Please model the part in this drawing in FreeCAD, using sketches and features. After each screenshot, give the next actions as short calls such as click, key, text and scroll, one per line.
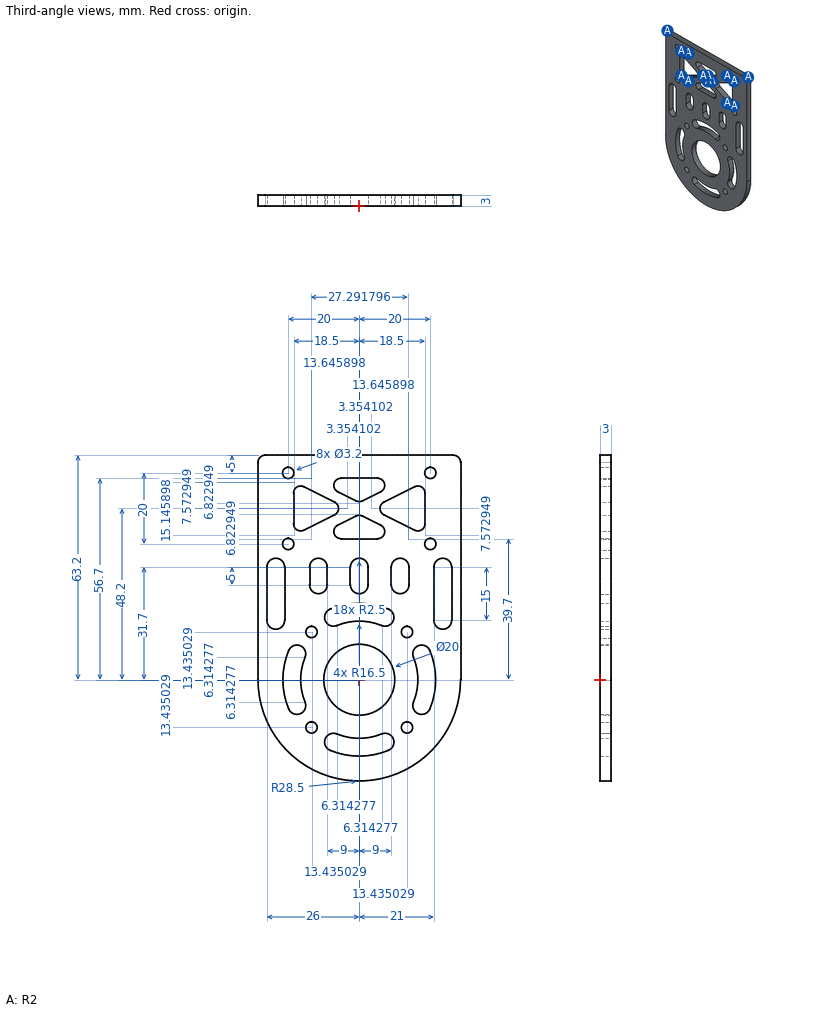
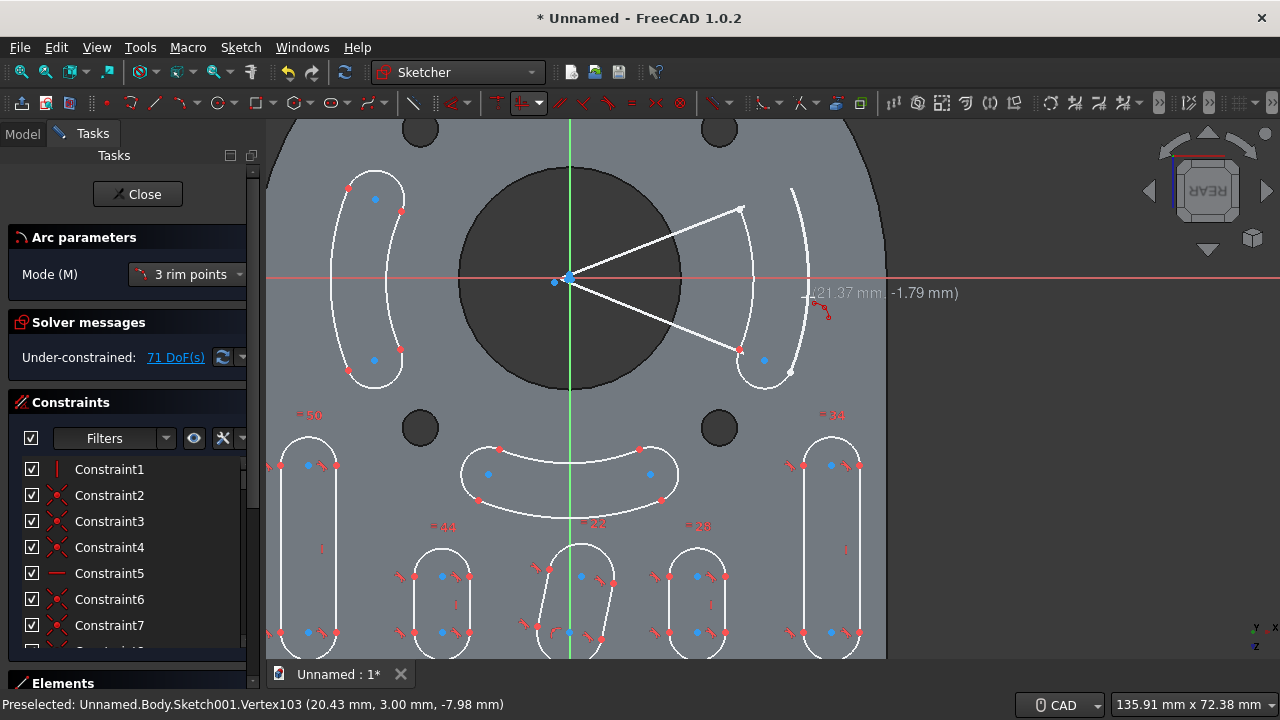
click(808, 297)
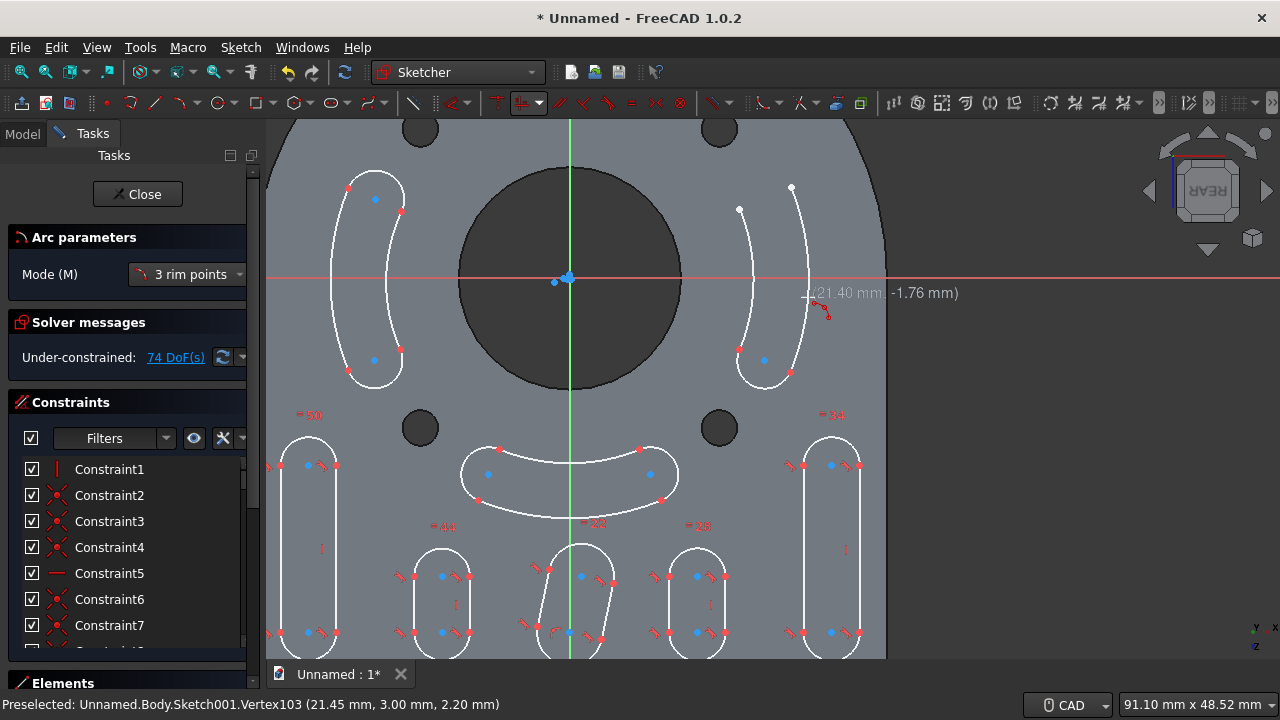
click(791, 188)
click(740, 209)
click(755, 172)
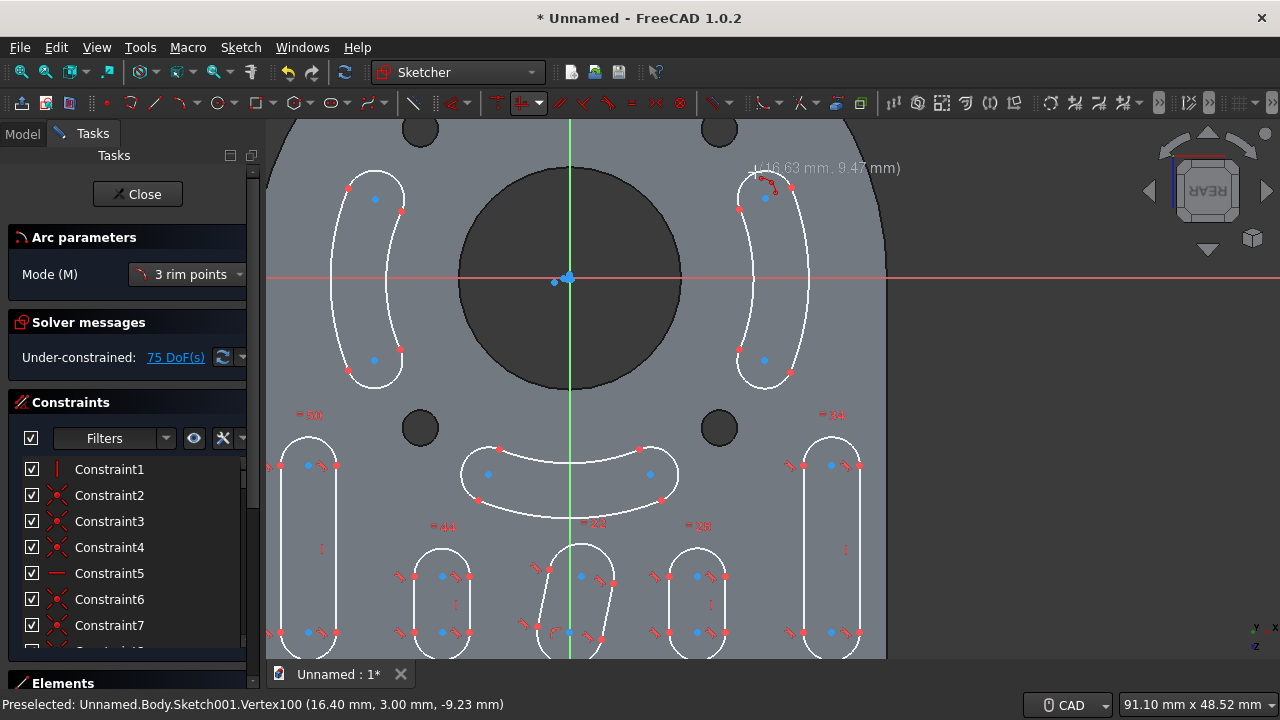
scroll(783, 339, down, 5)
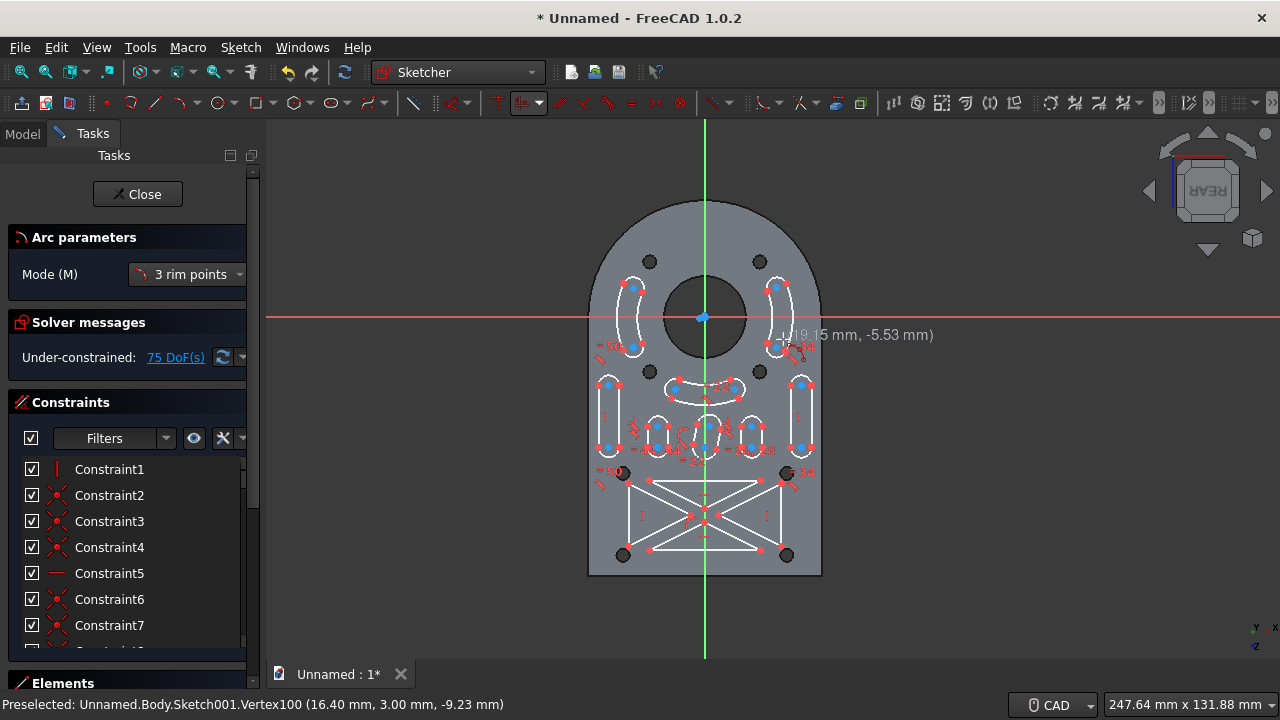
click(679, 255)
click(731, 255)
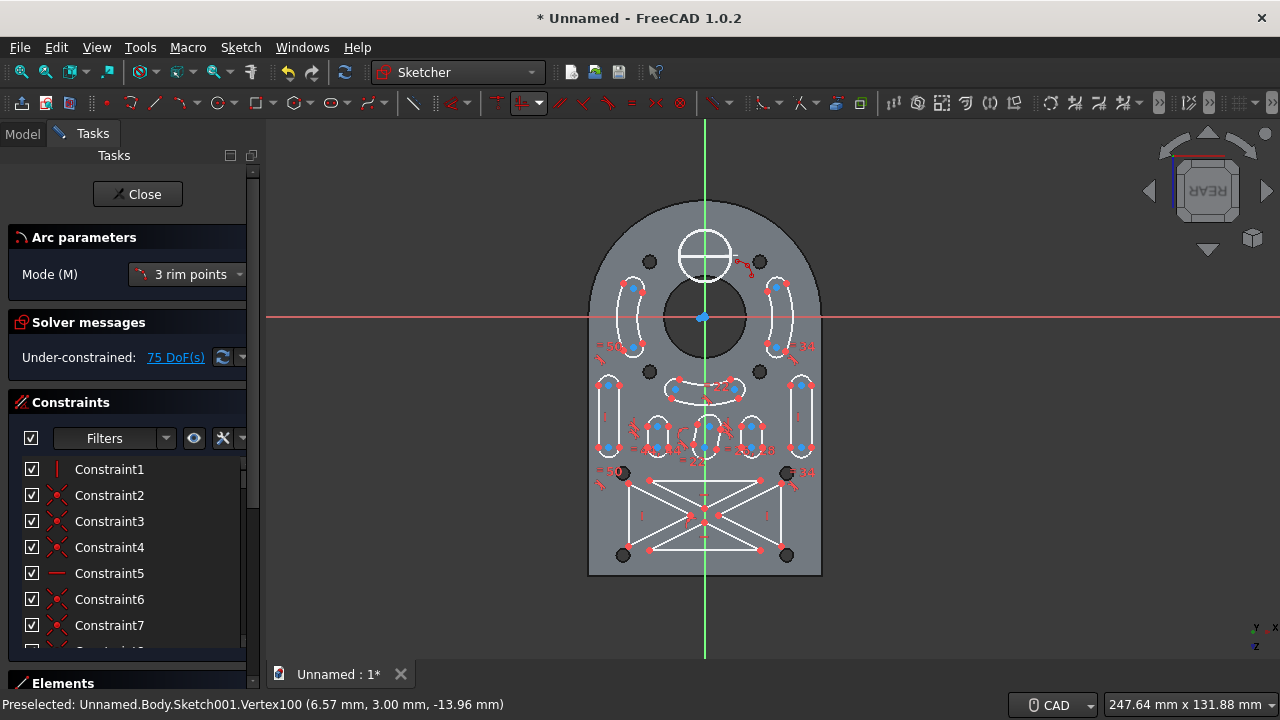
scroll(710, 250, up, 6)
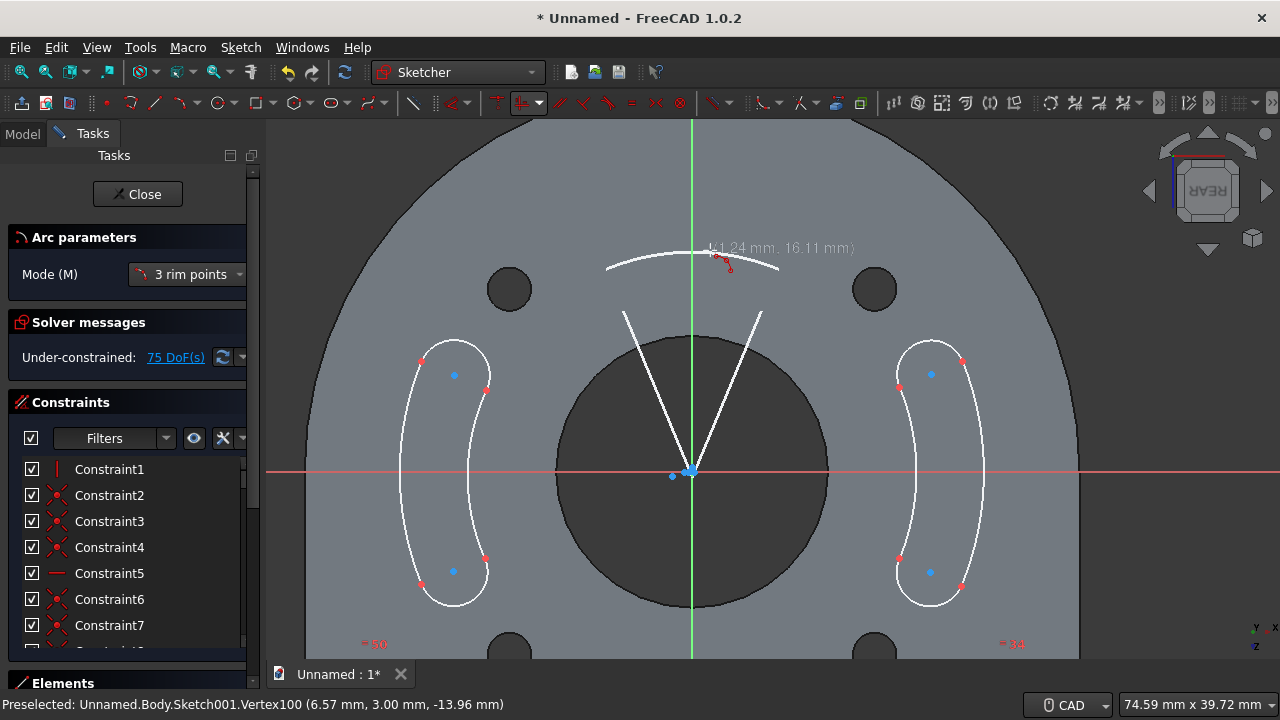
click(710, 248)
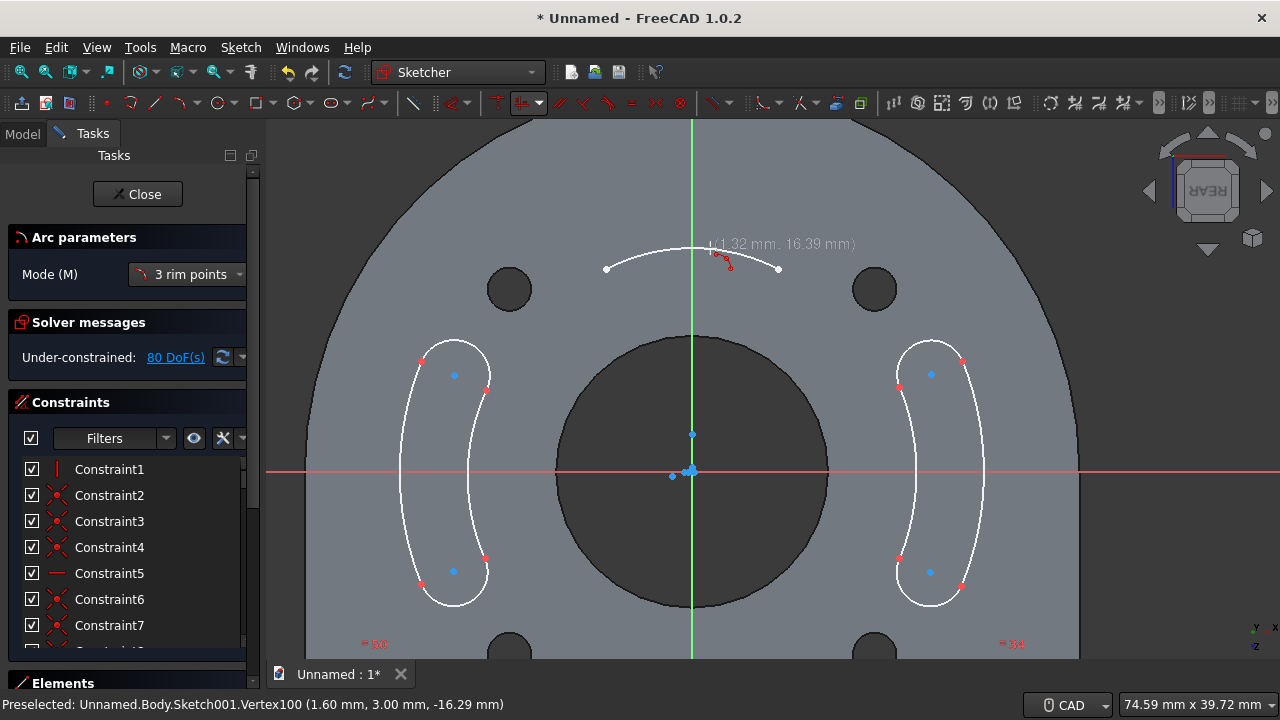
click(779, 269)
click(804, 202)
click(822, 246)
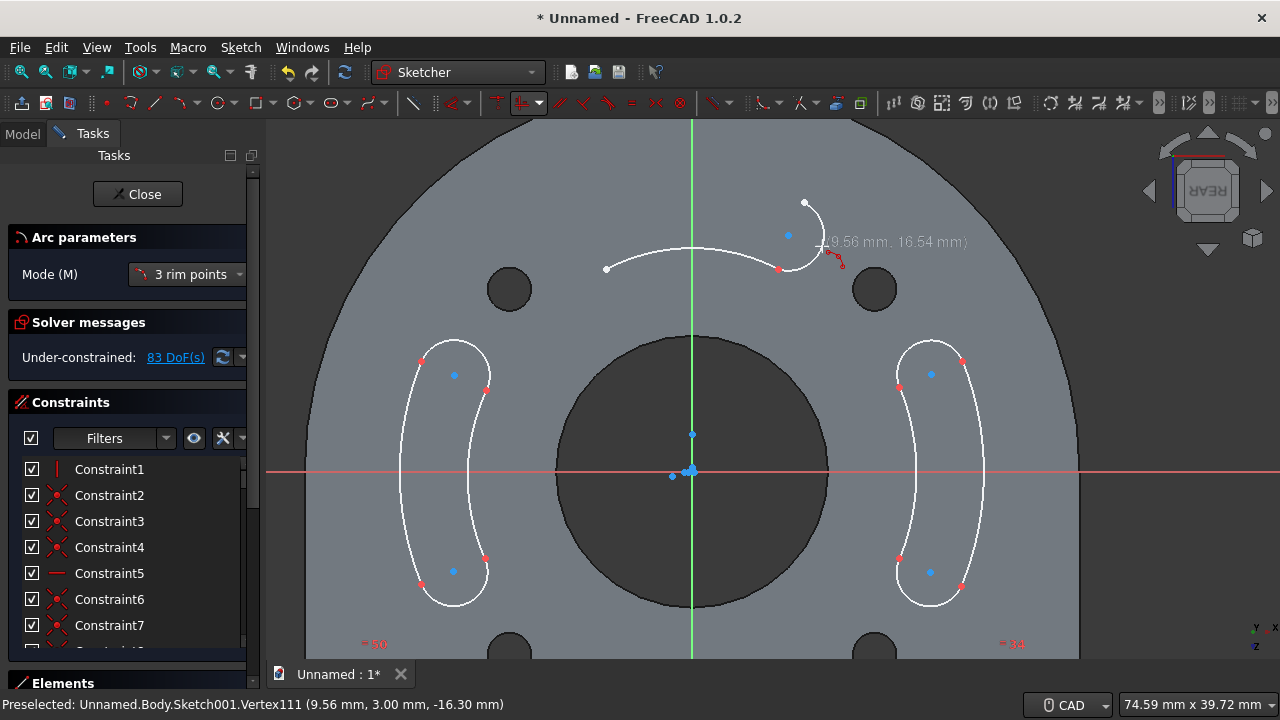
click(804, 203)
click(580, 202)
click(715, 180)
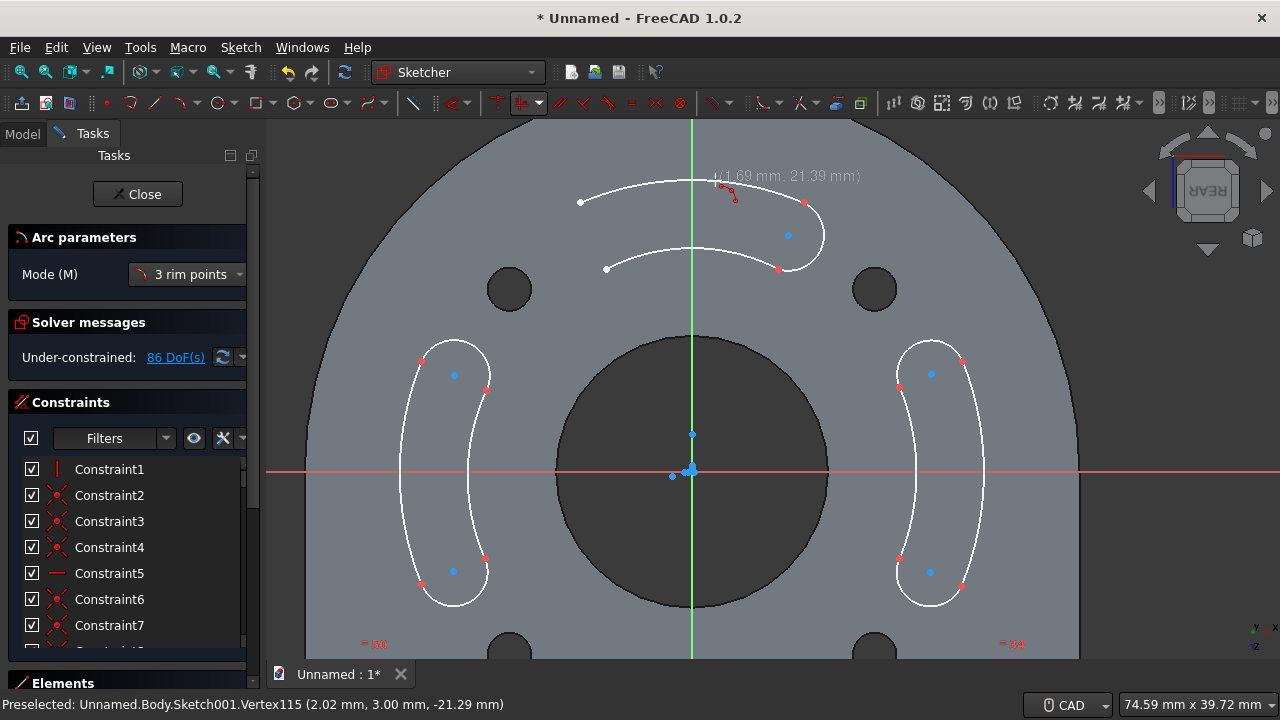
click(580, 203)
click(606, 269)
click(562, 246)
key(Escape)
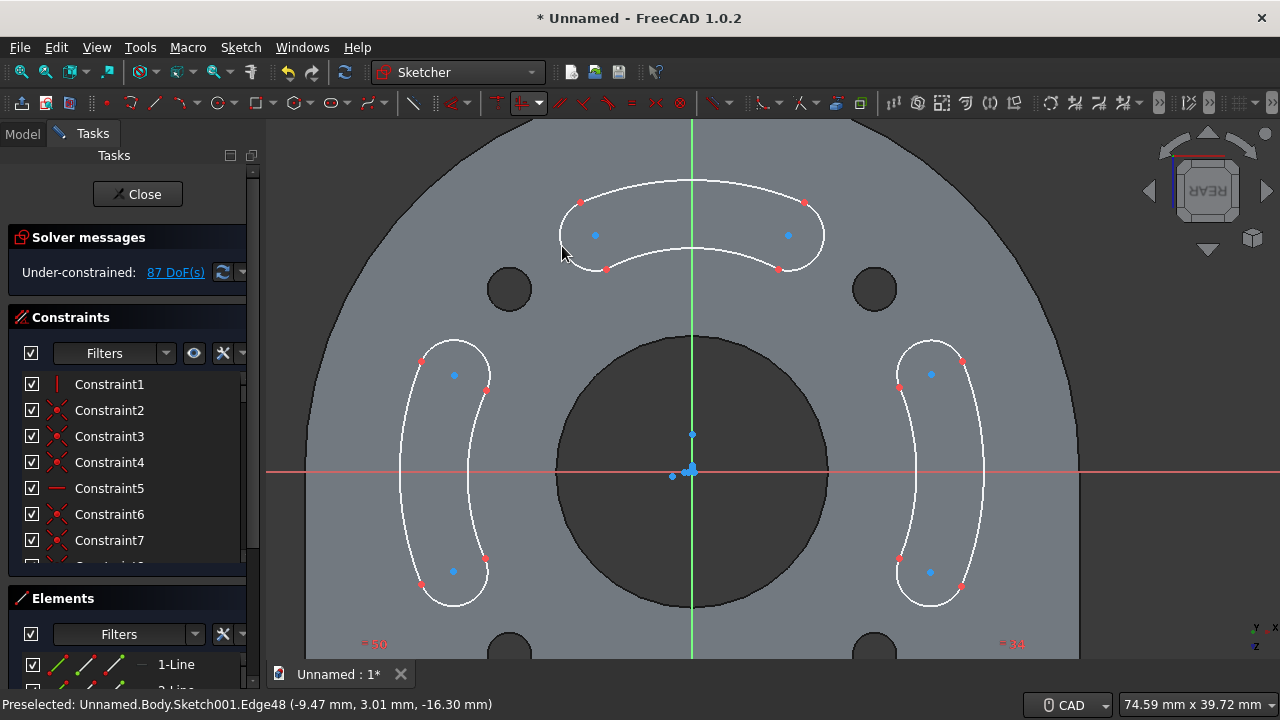
scroll(710, 250, down, 6)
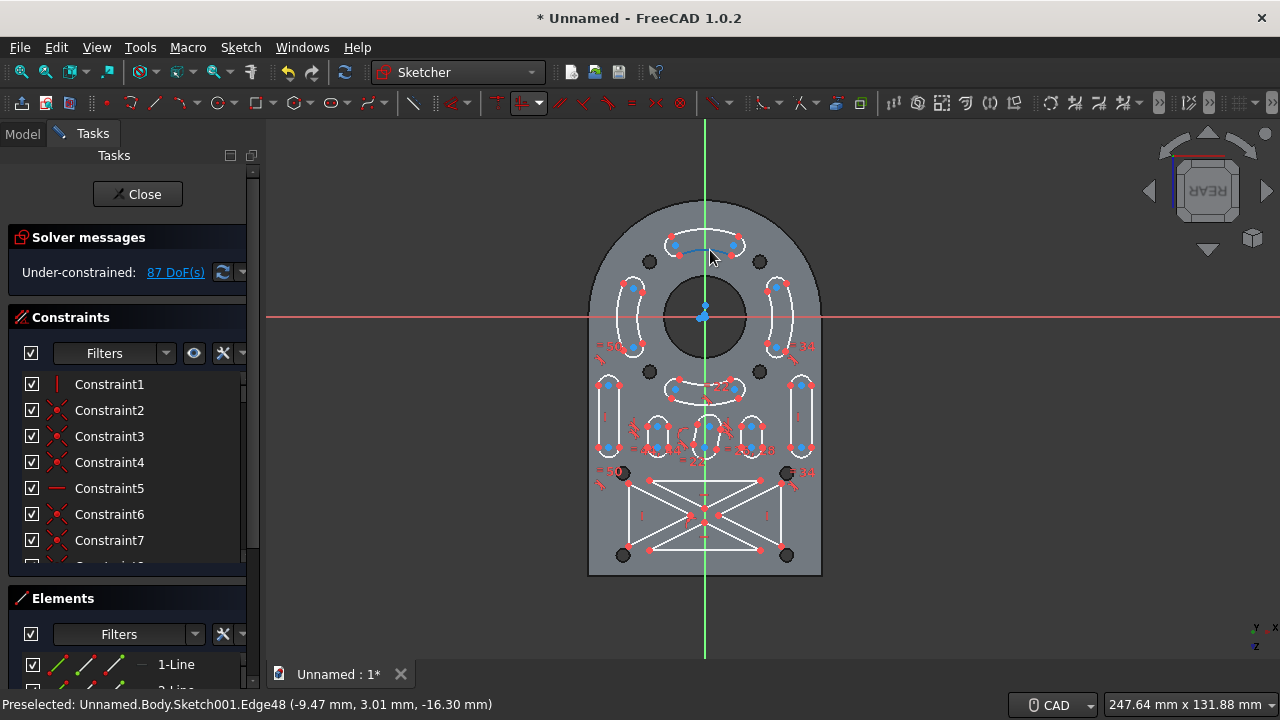
scroll(694, 384, up, 2)